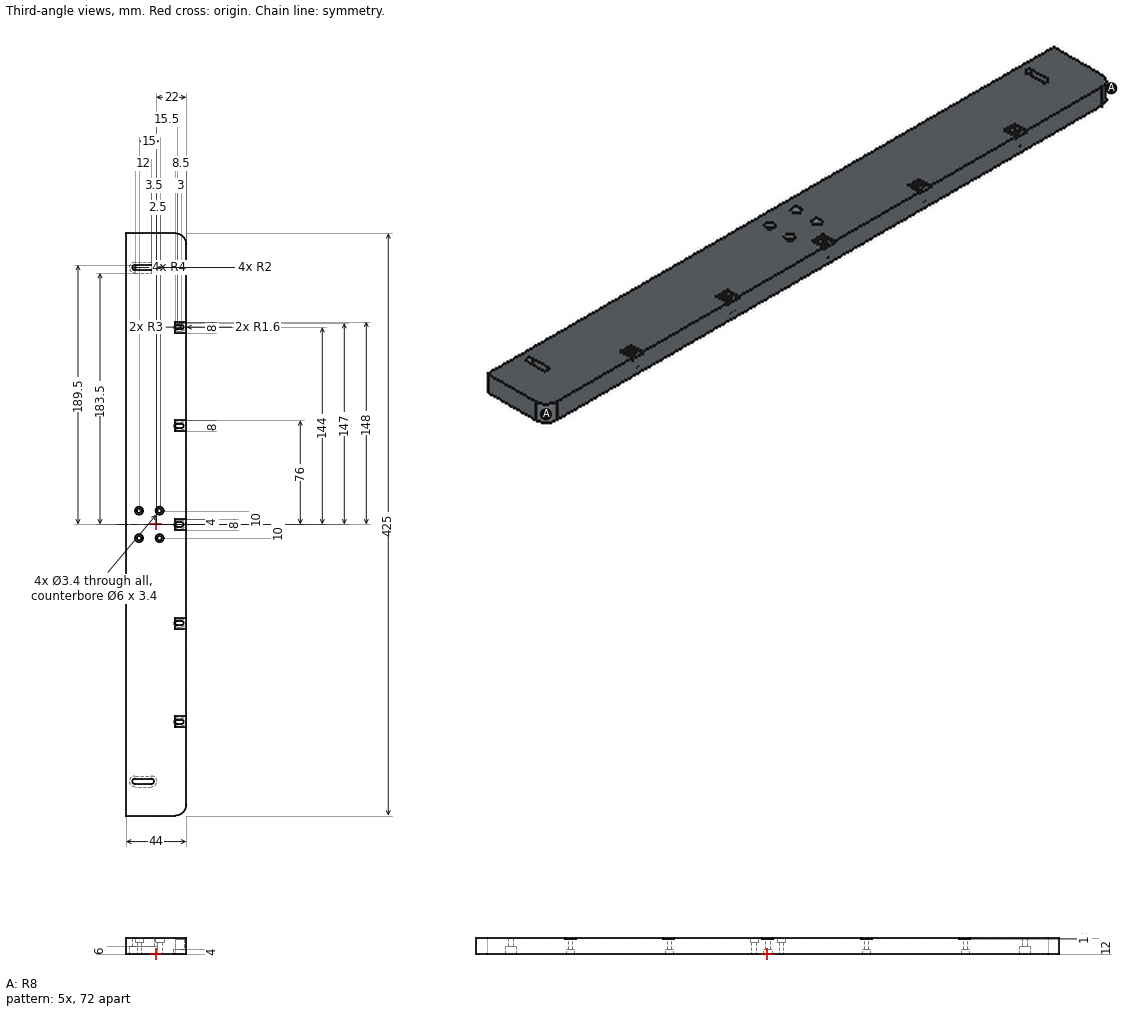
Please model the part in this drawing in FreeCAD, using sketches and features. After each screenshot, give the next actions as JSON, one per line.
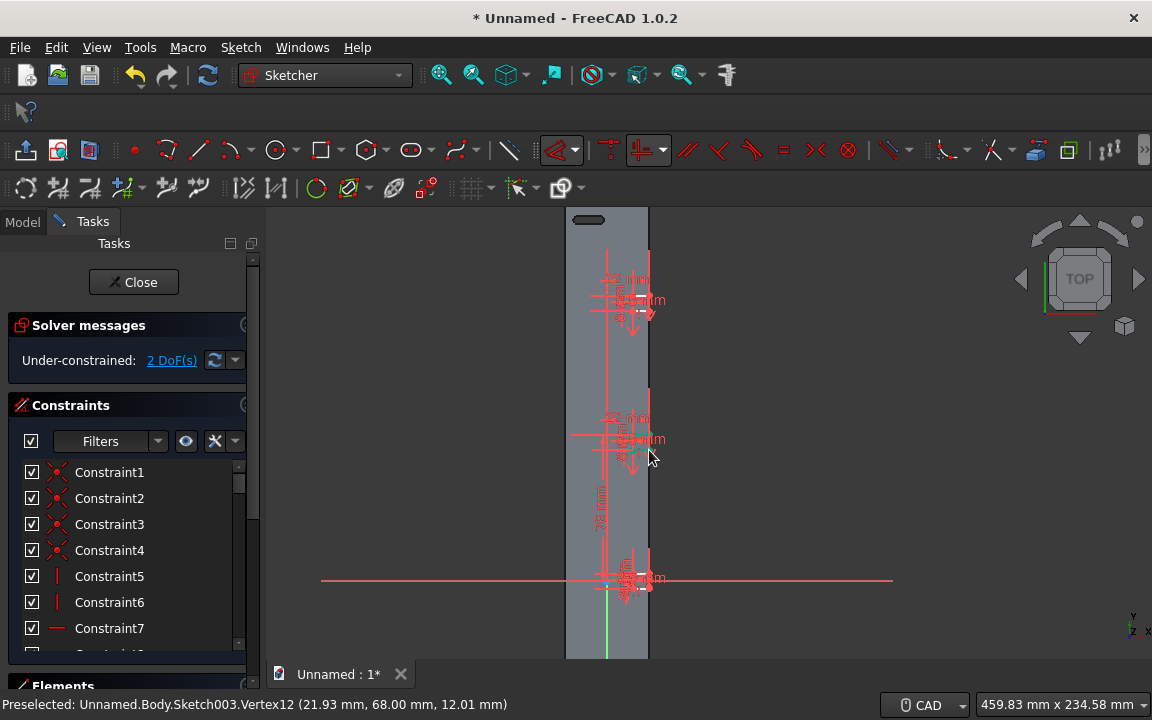
{"action": "left_click", "coordinate": [649, 589]}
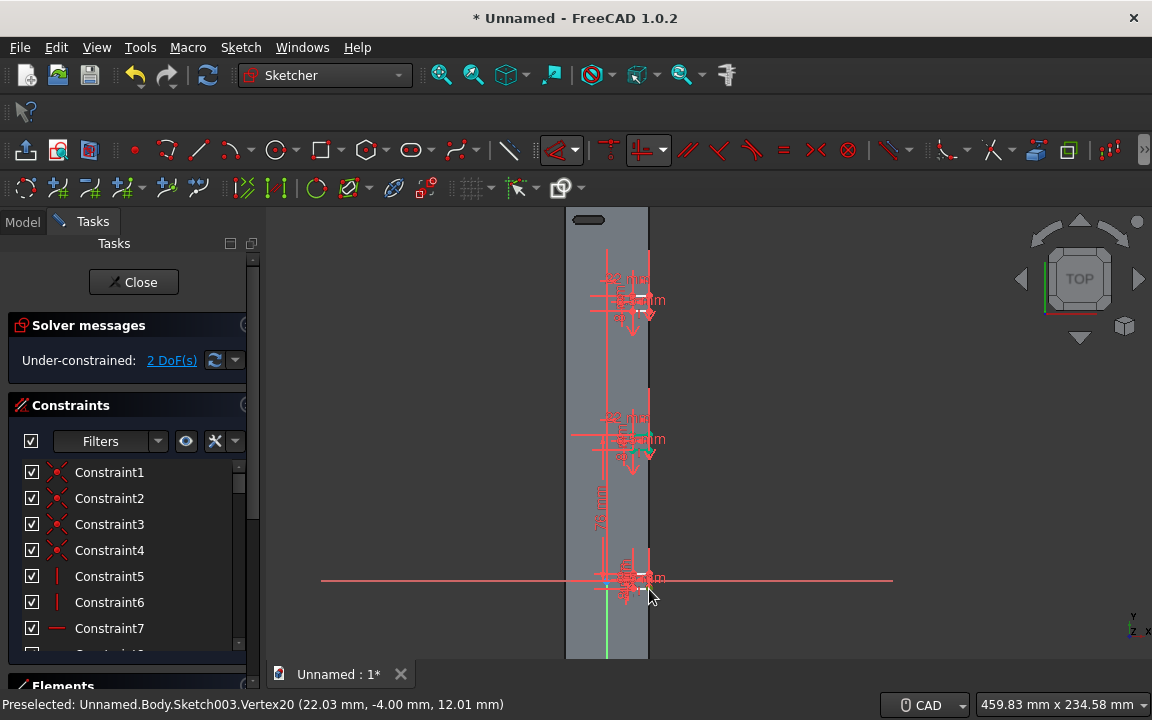
{"action": "key", "text": "l"}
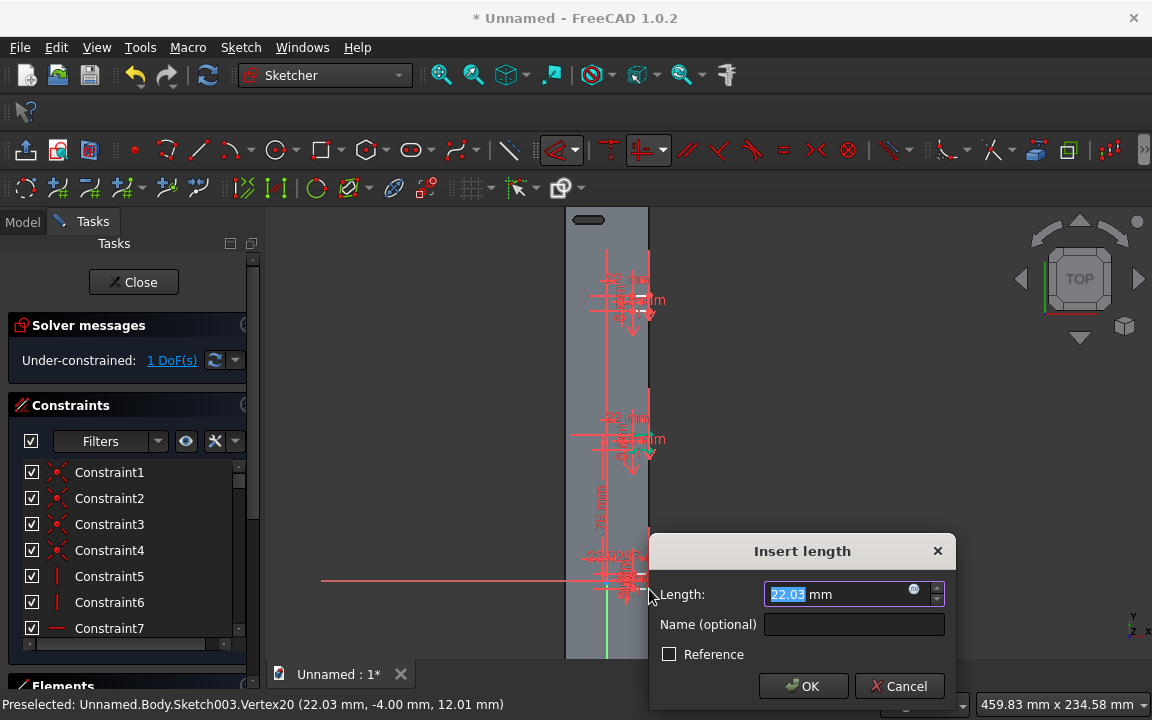
{"action": "type", "text": "22"}
{"action": "key", "text": "Return"}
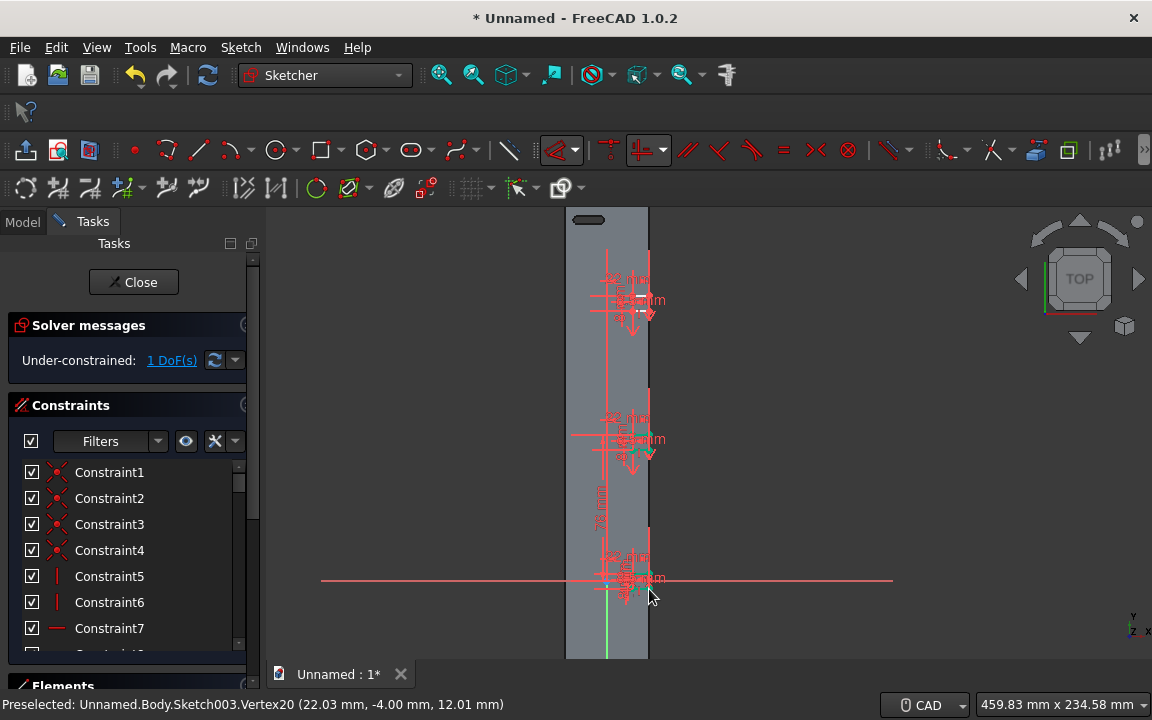
{"action": "left_click", "coordinate": [633, 296]}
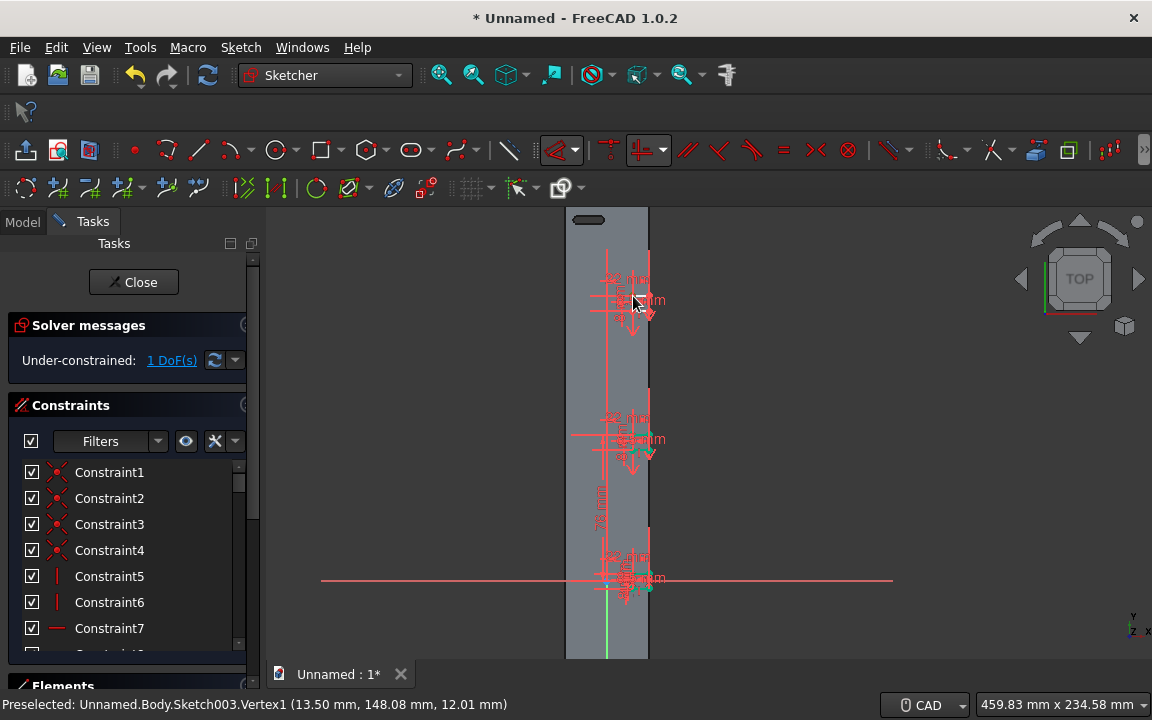
{"action": "key", "text": "i"}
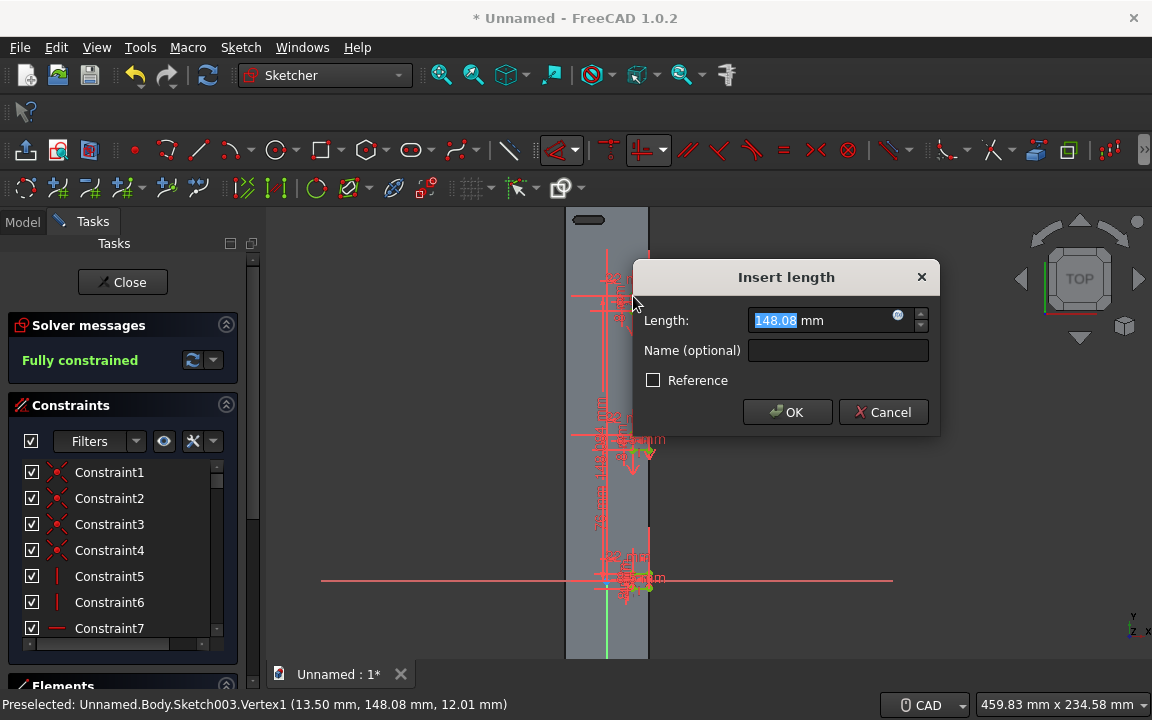
{"action": "type", "text": "148"}
{"action": "key", "text": "Return"}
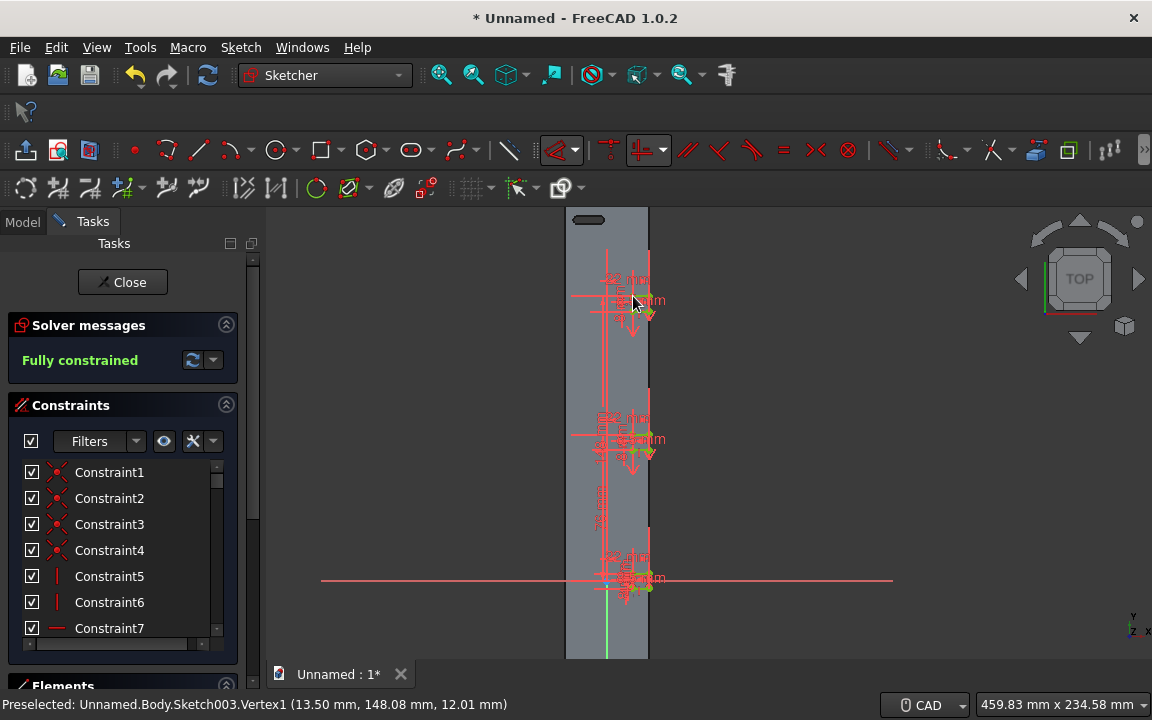
{"action": "left_click", "coordinate": [123, 282]}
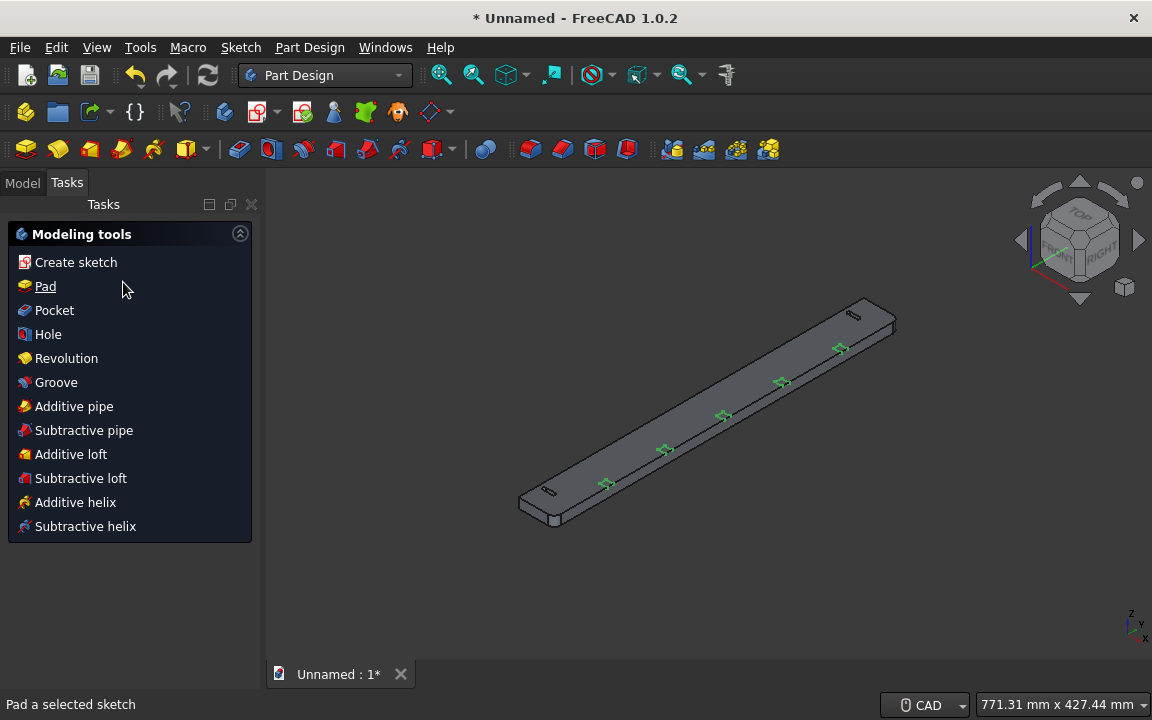
{"action": "left_click", "coordinate": [240, 150]}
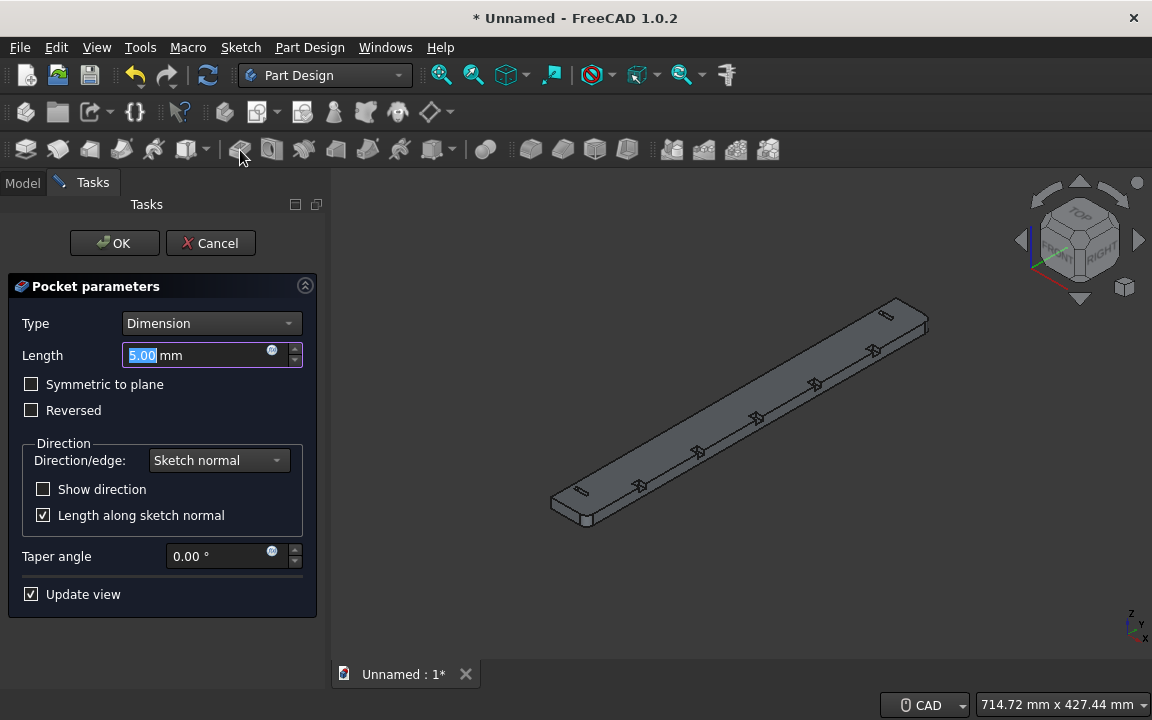
{"action": "type", "text": "1"}
{"action": "key", "text": "Tab"}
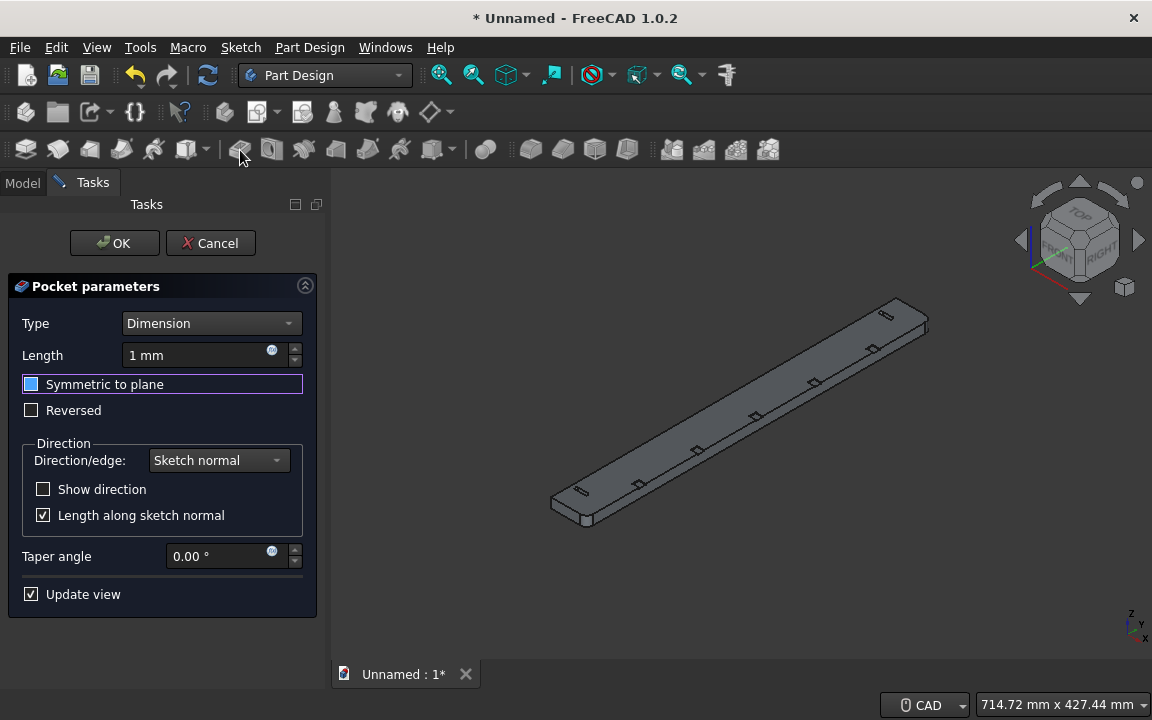
{"action": "left_click", "coordinate": [115, 243]}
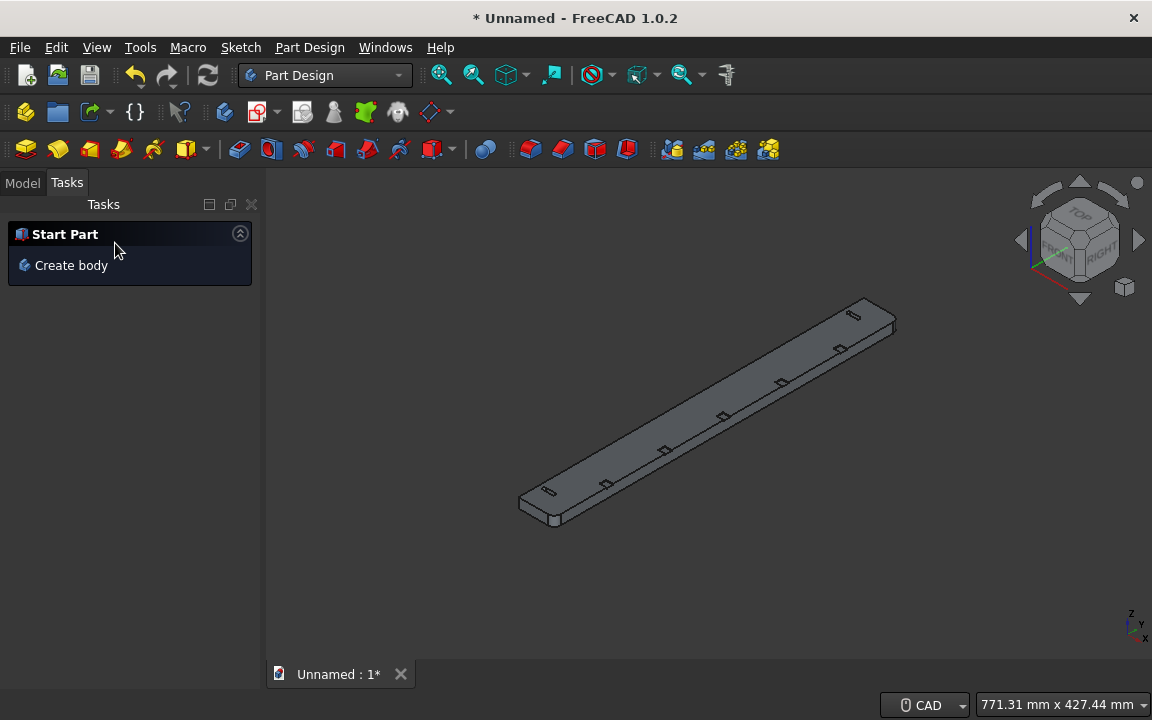
{"action": "left_click", "coordinate": [258, 112]}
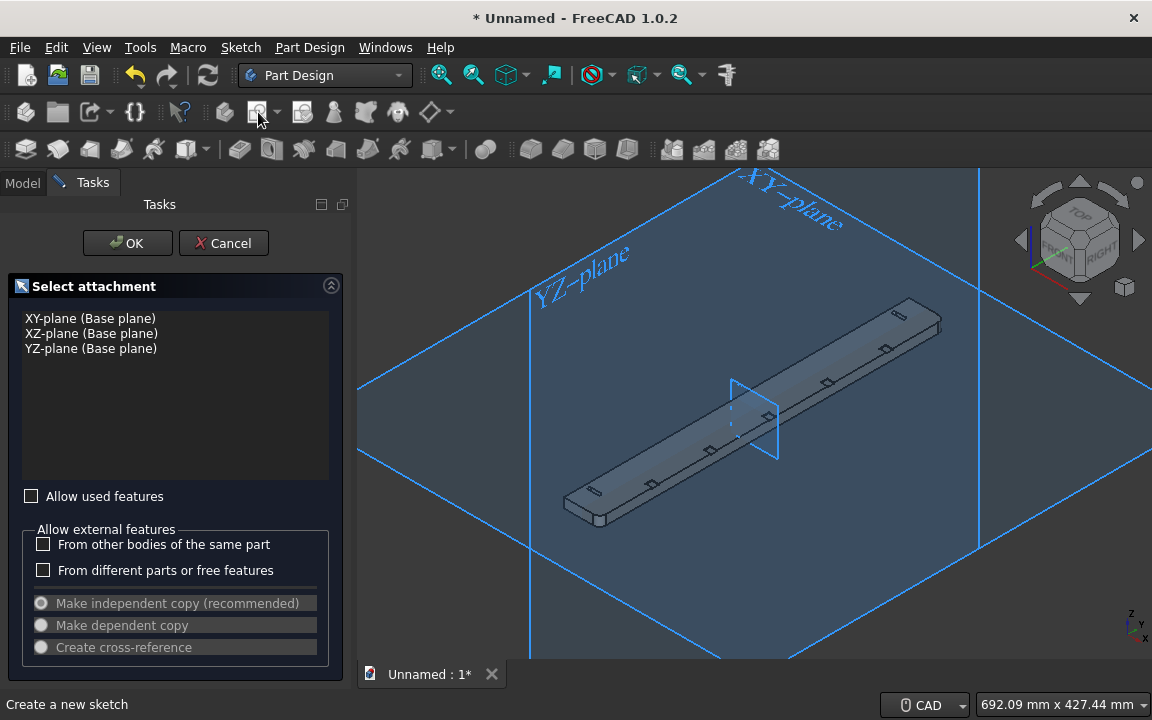
{"action": "left_click", "coordinate": [82, 318]}